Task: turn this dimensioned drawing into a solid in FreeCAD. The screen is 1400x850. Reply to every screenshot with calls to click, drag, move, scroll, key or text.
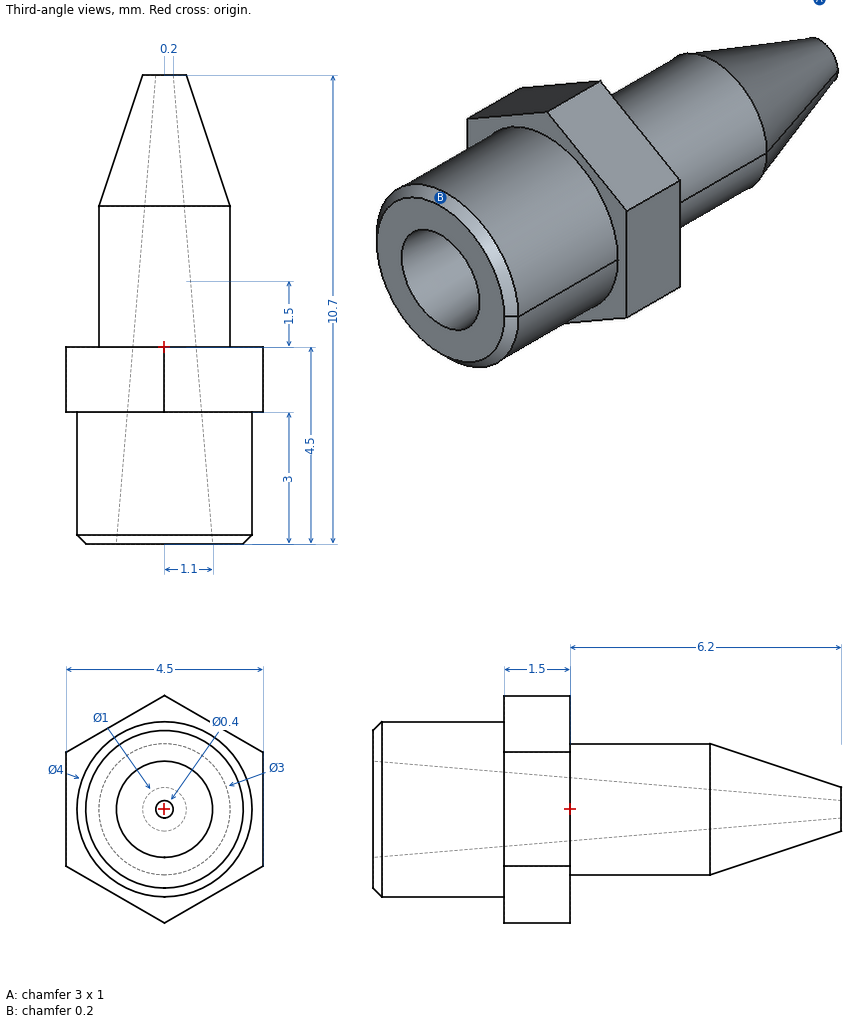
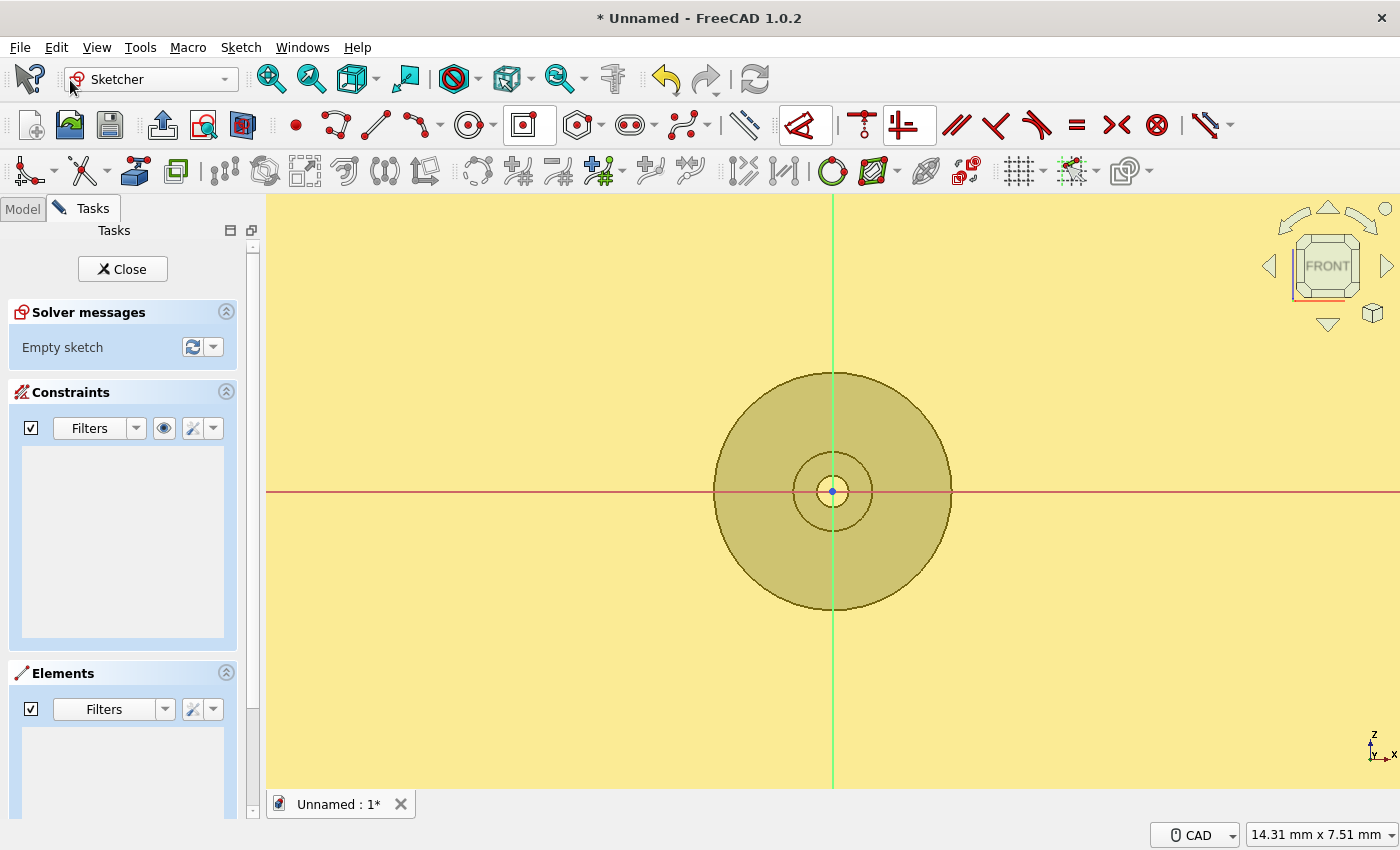
click(578, 126)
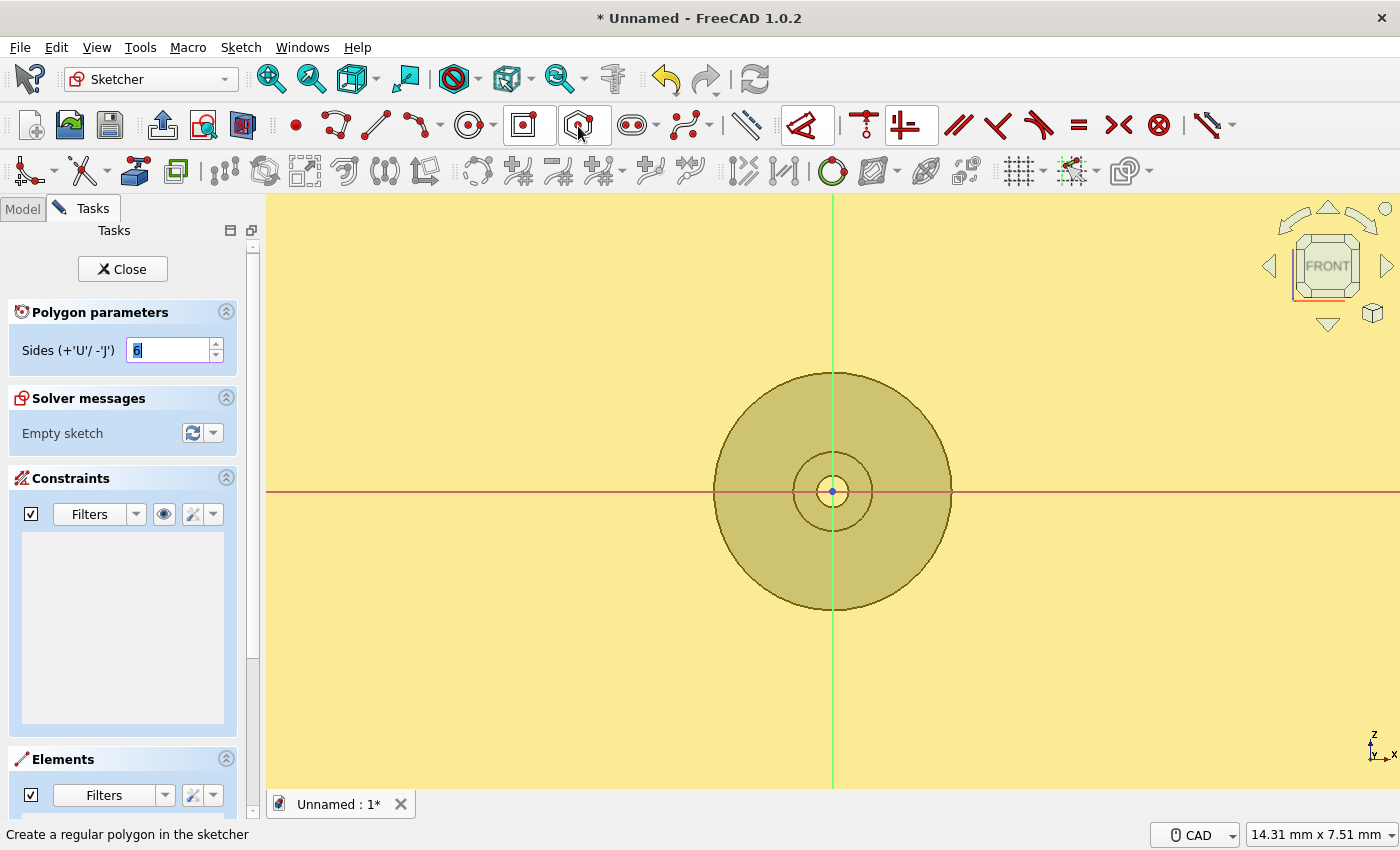
click(833, 492)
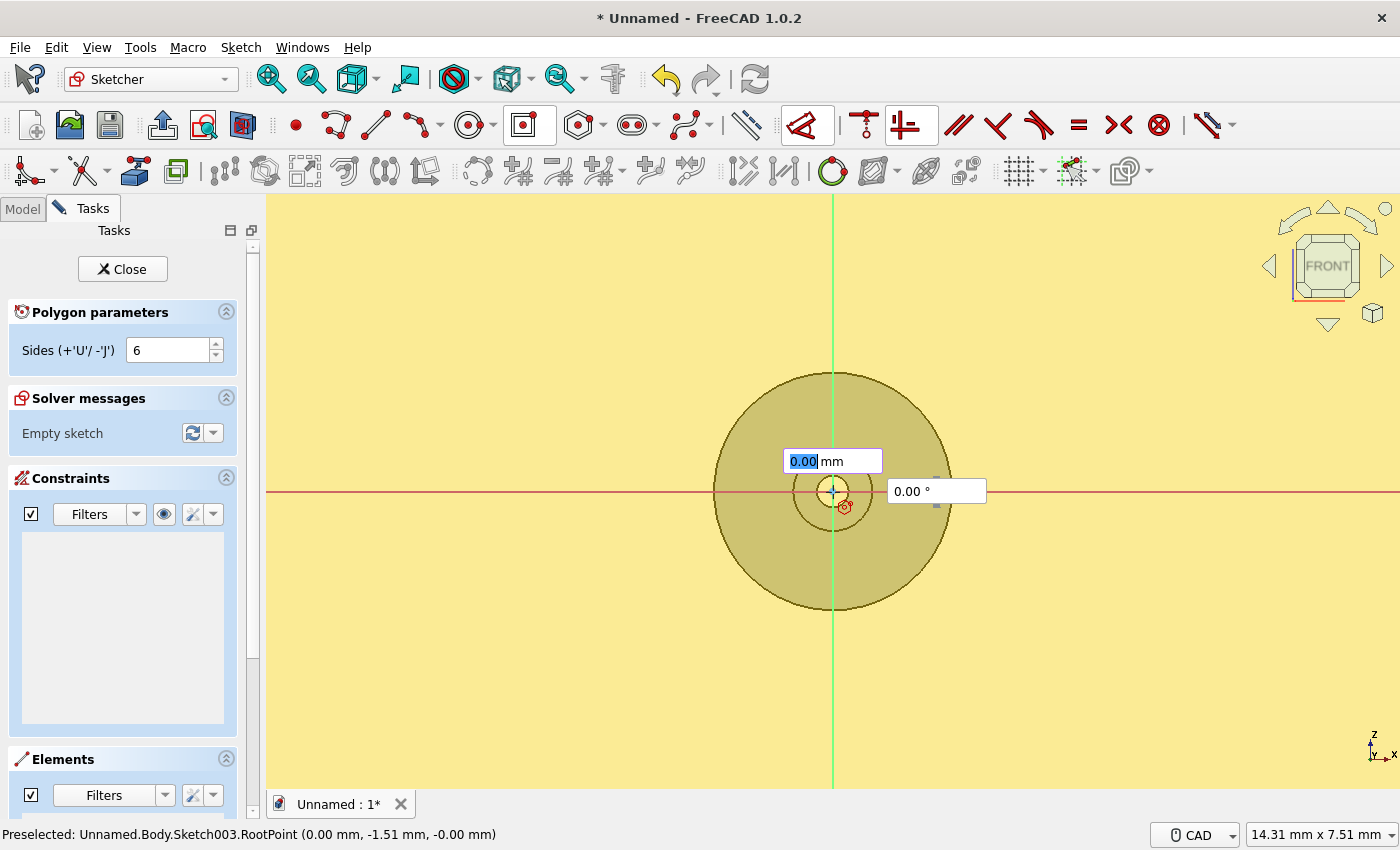
click(833, 286)
right_click(833, 286)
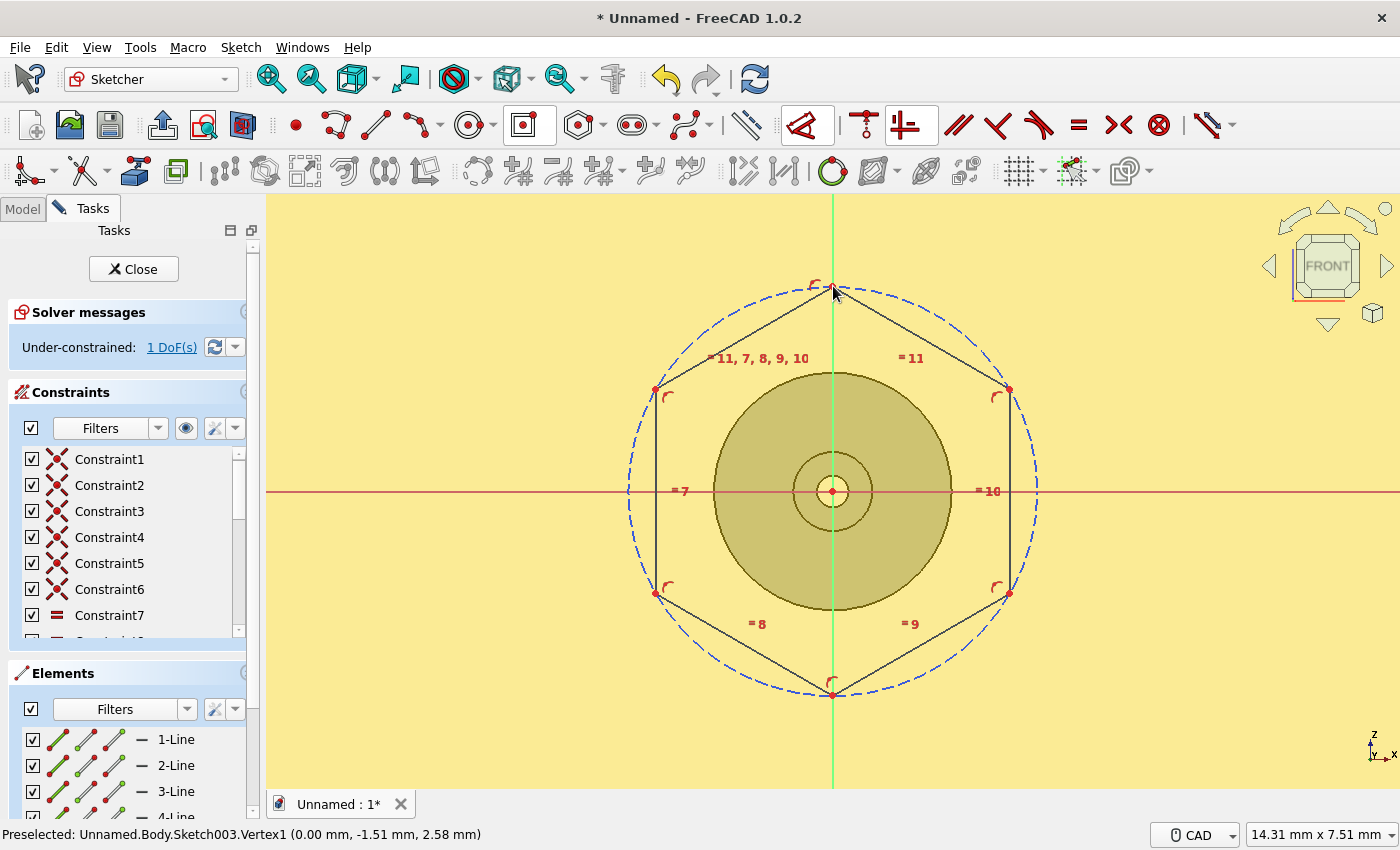
click(470, 126)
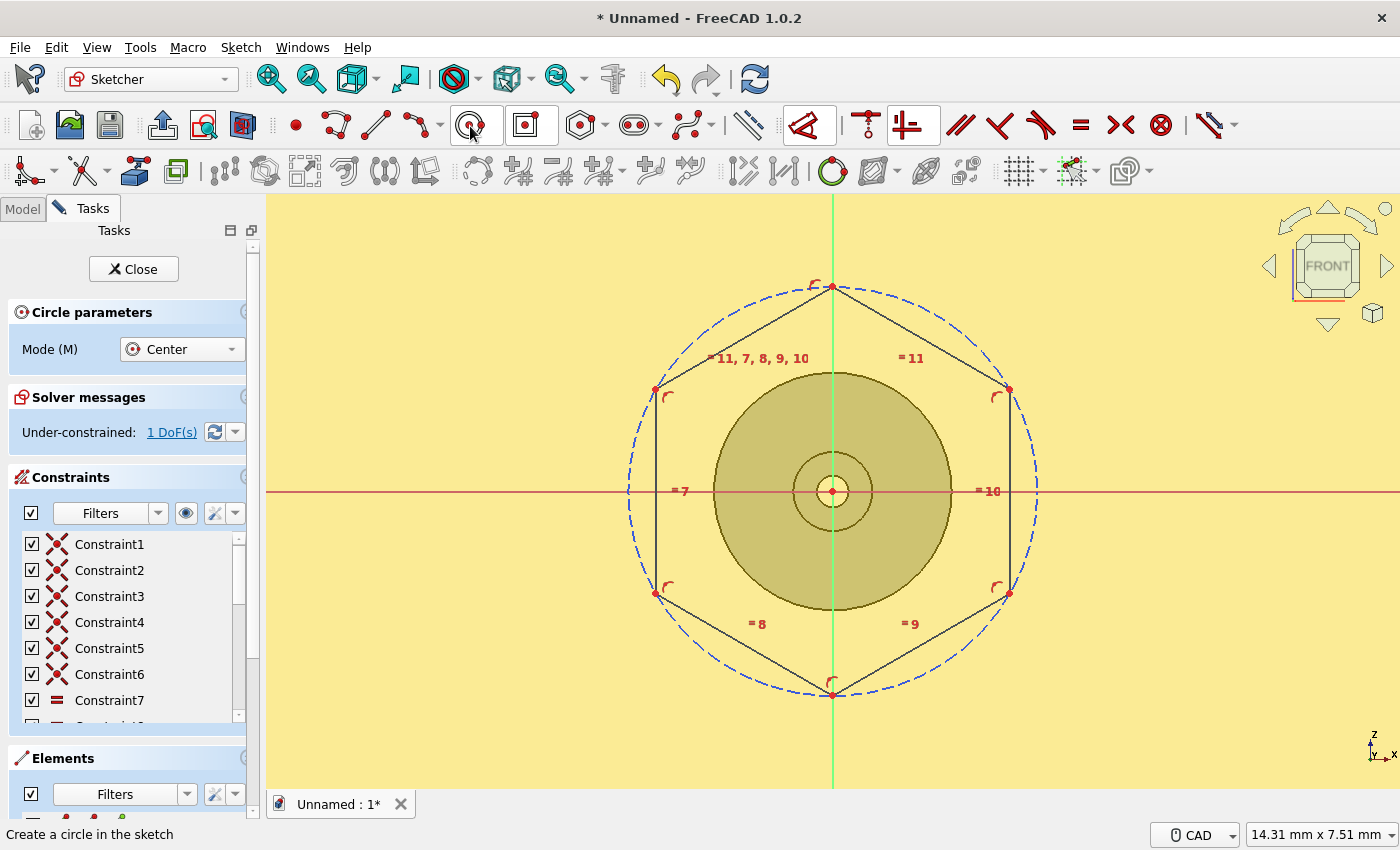
click(833, 492)
click(861, 463)
key(Escape)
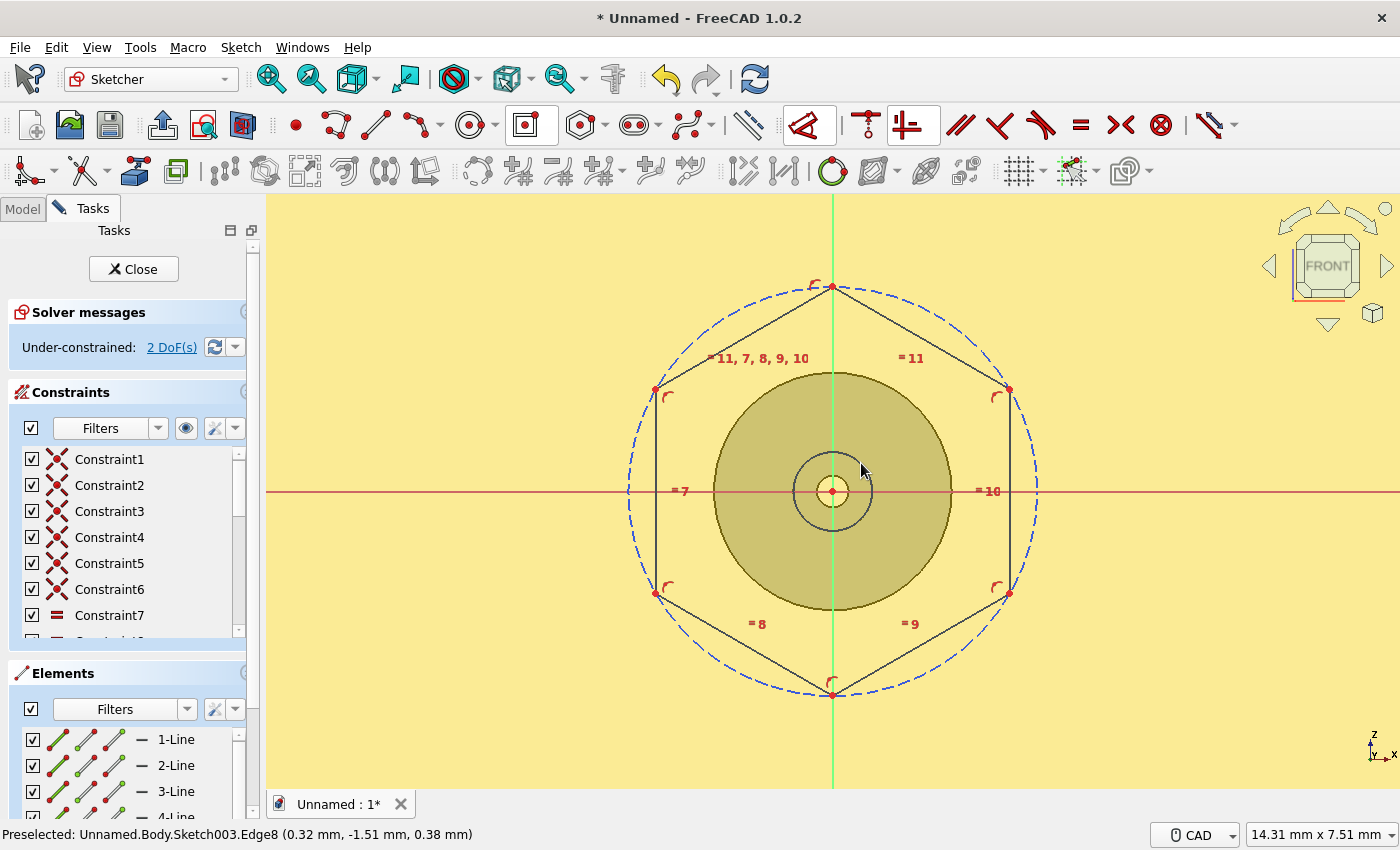
click(861, 464)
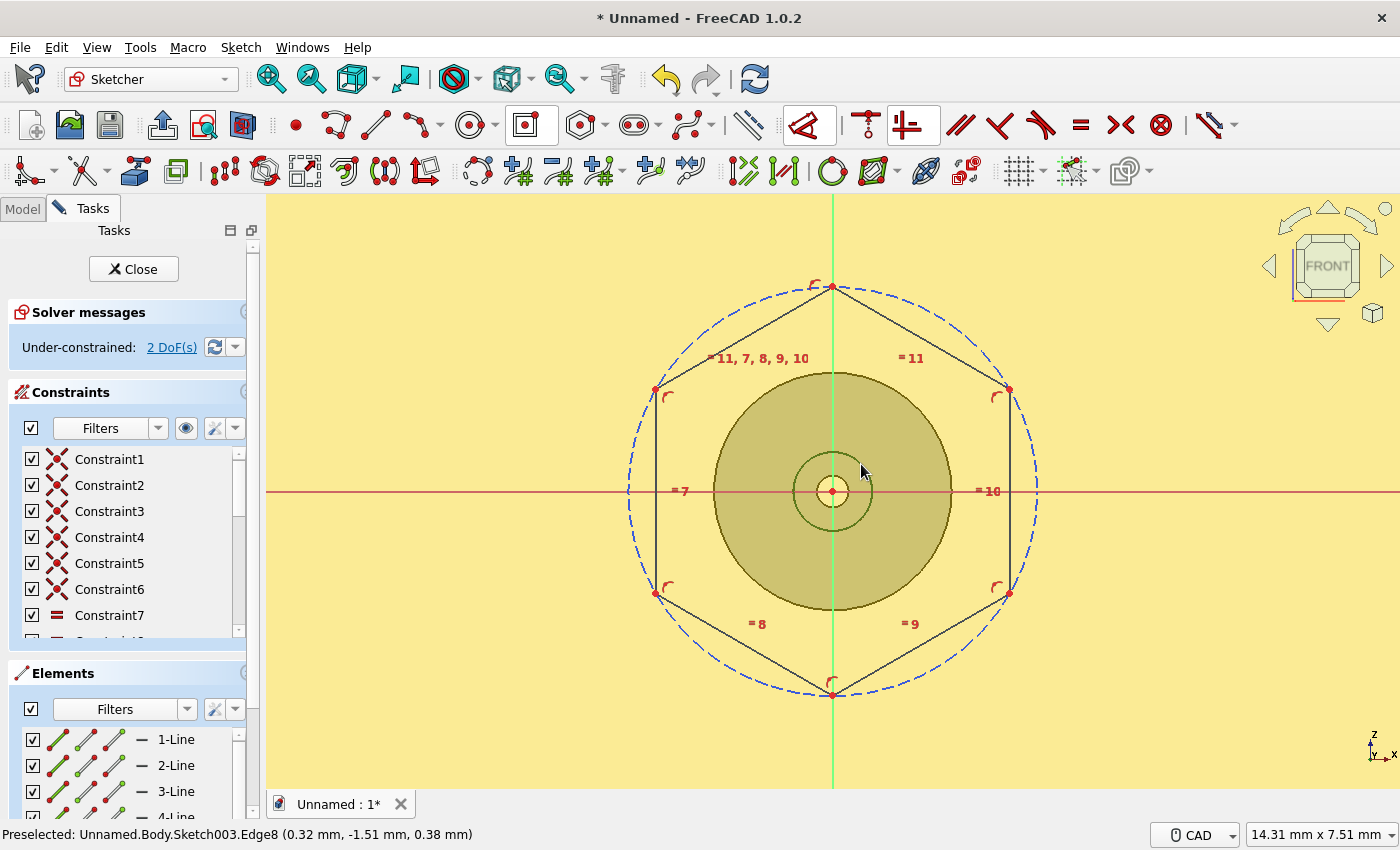
click(830, 126)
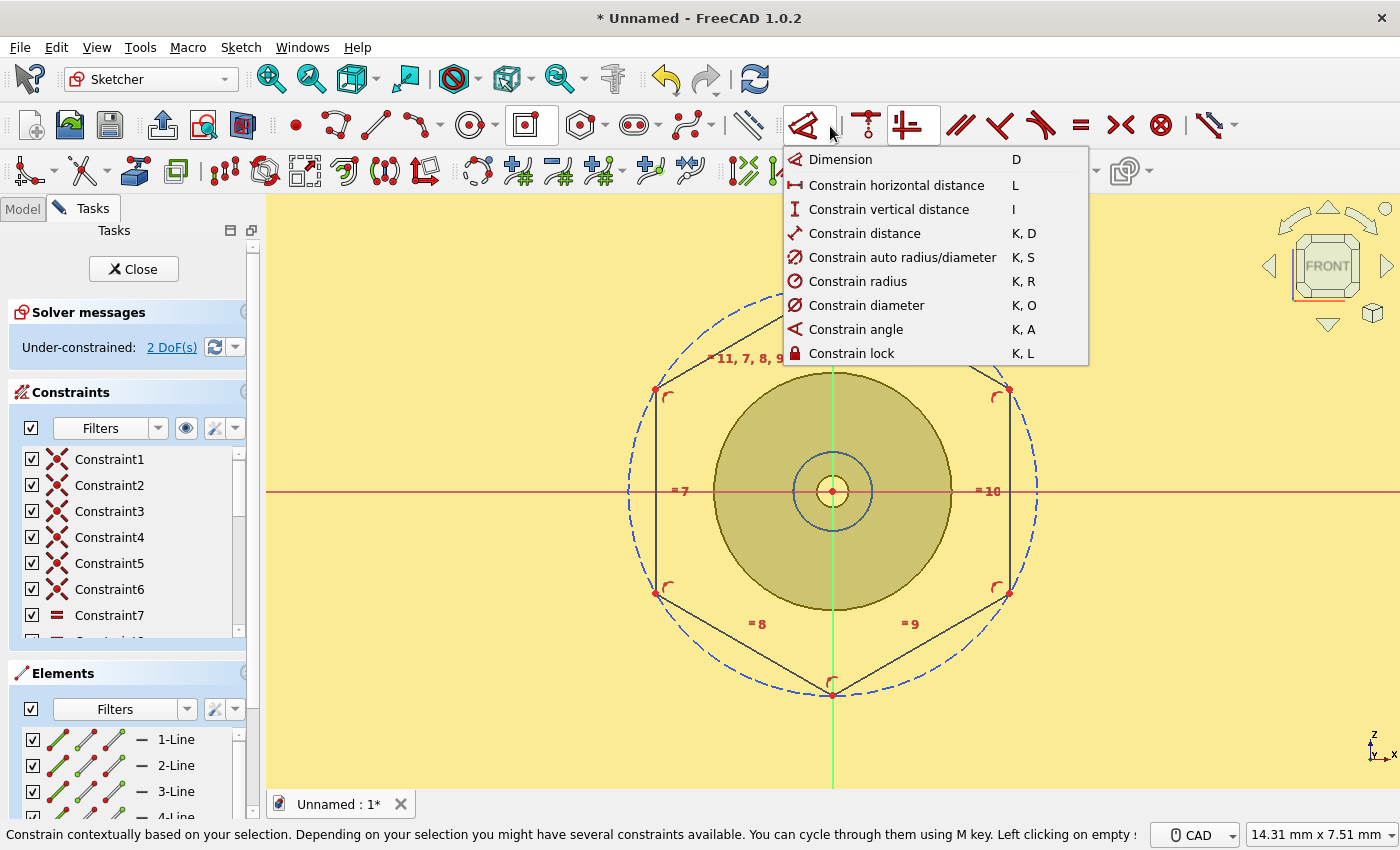
click(936, 305)